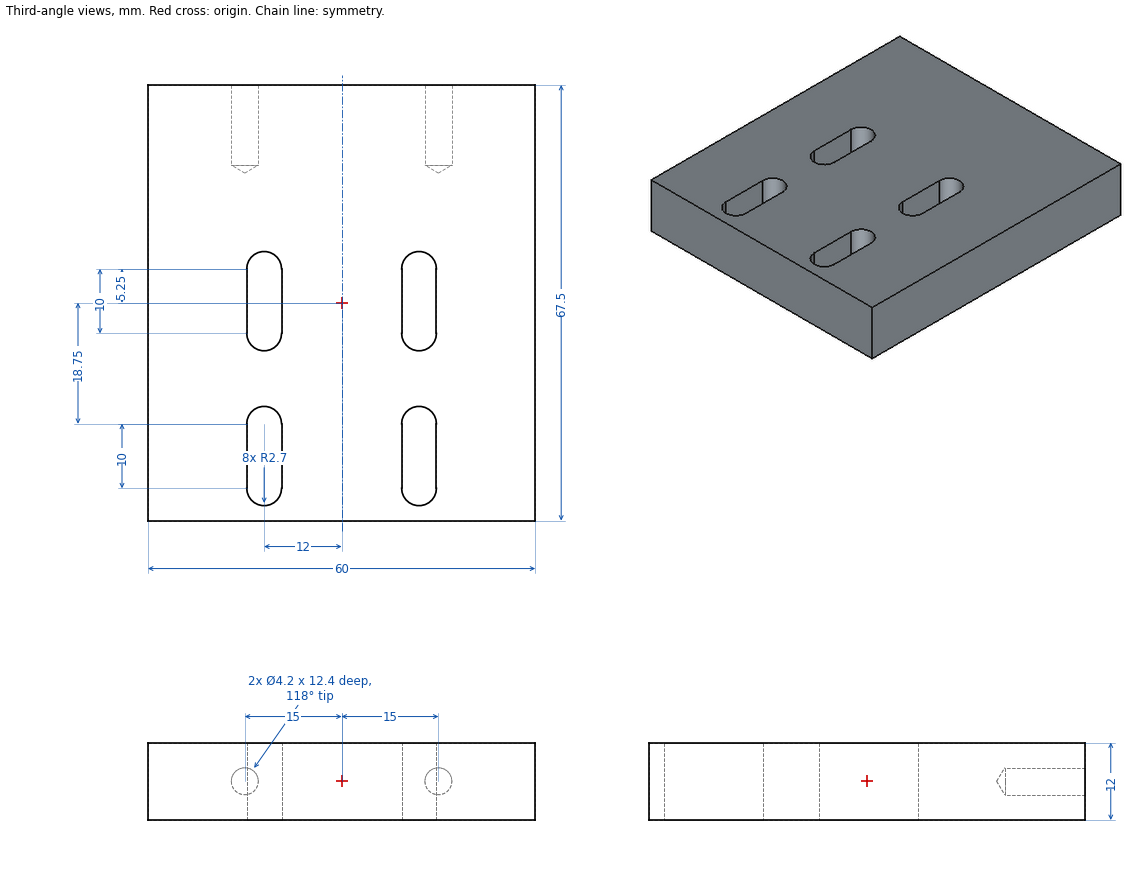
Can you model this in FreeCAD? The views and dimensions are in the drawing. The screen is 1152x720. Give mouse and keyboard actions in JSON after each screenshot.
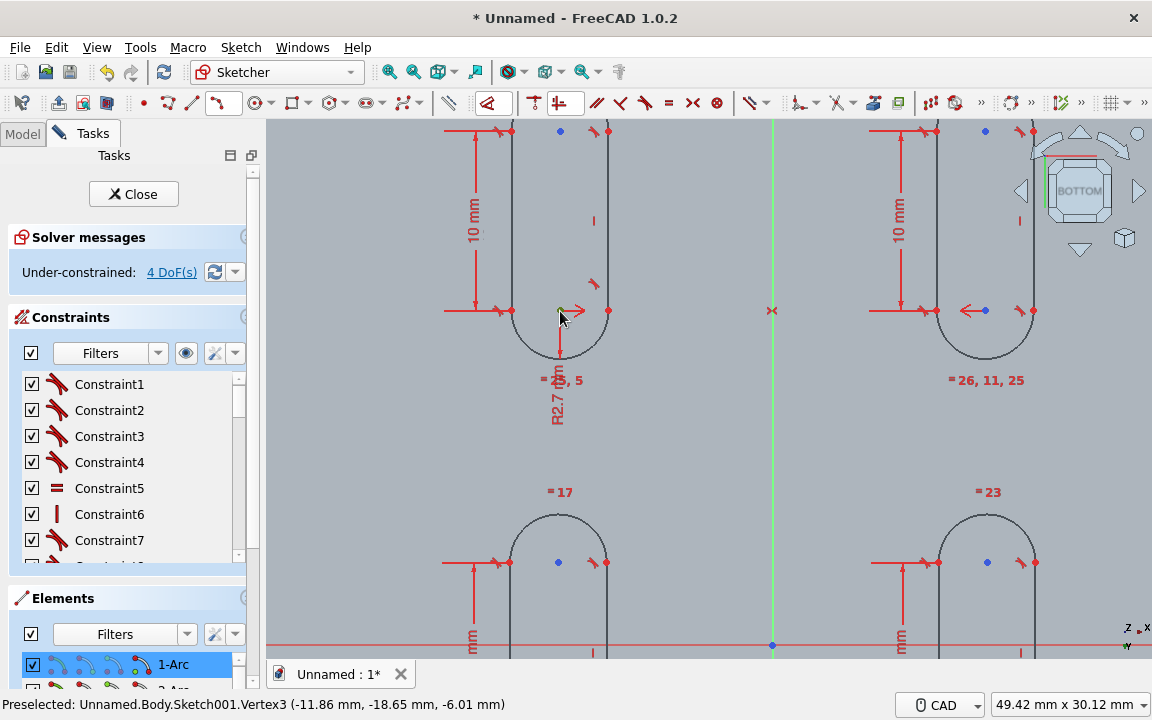
{"action": "key", "text": "l"}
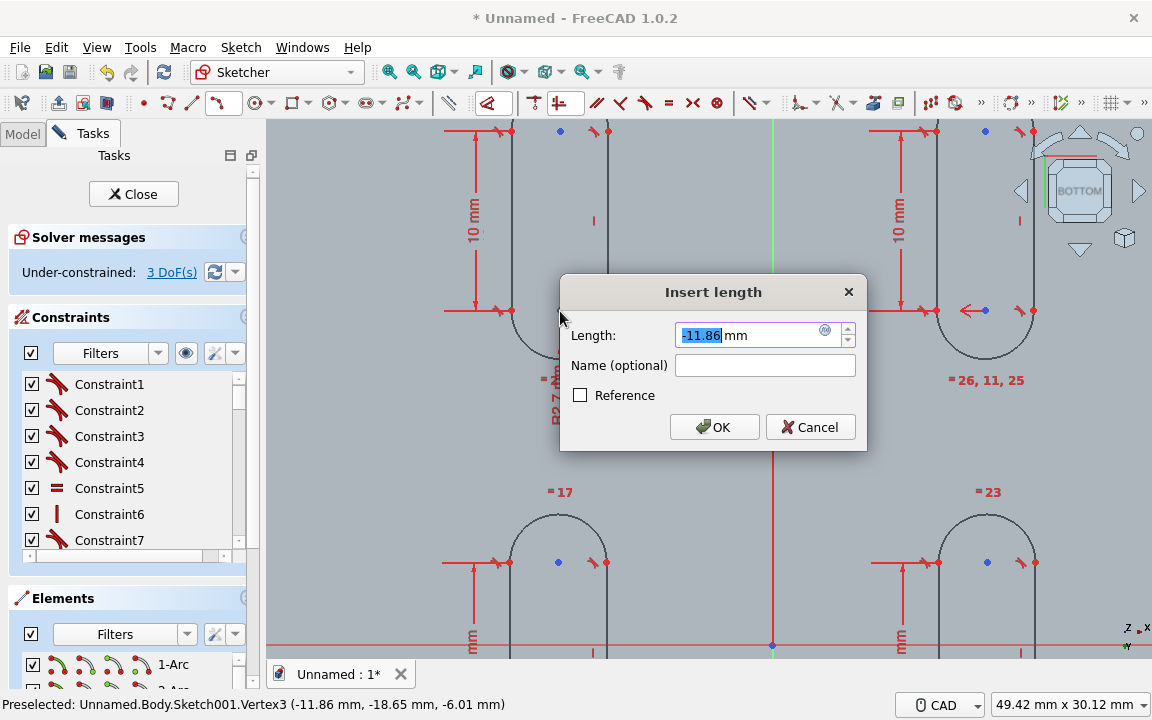
{"action": "type", "text": "-12"}
{"action": "key", "text": "Return"}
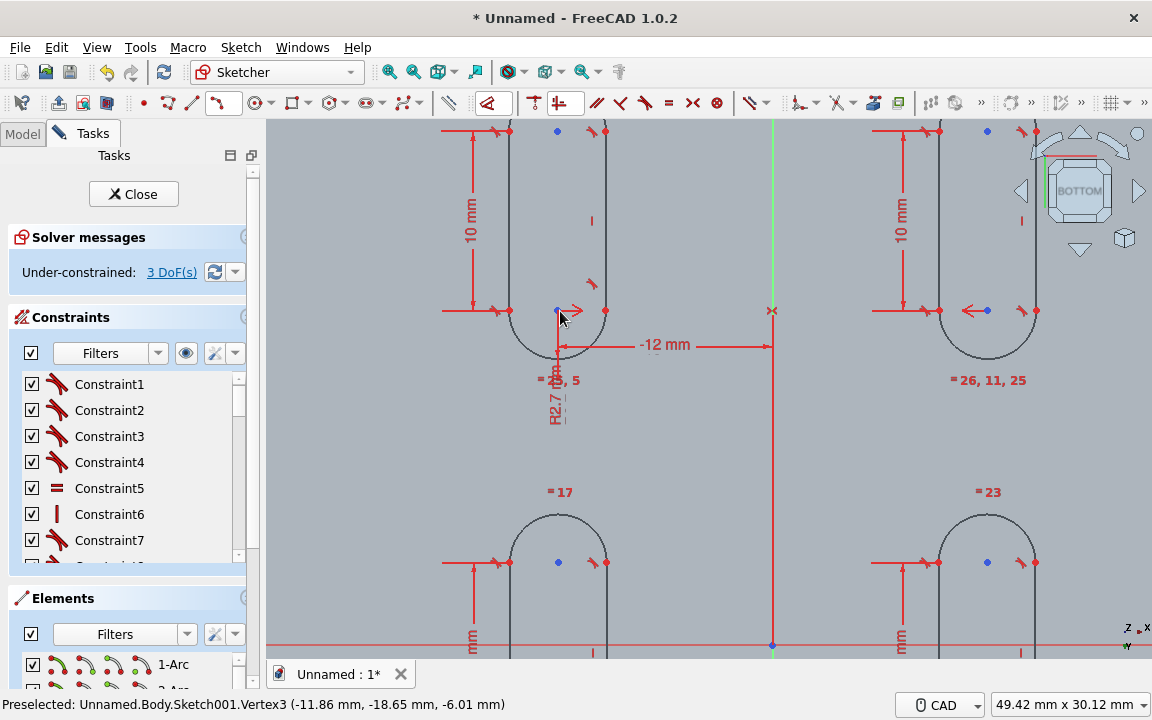
{"action": "scroll", "coordinate": [533, 352], "scroll_direction": "down", "scroll_amount": 4}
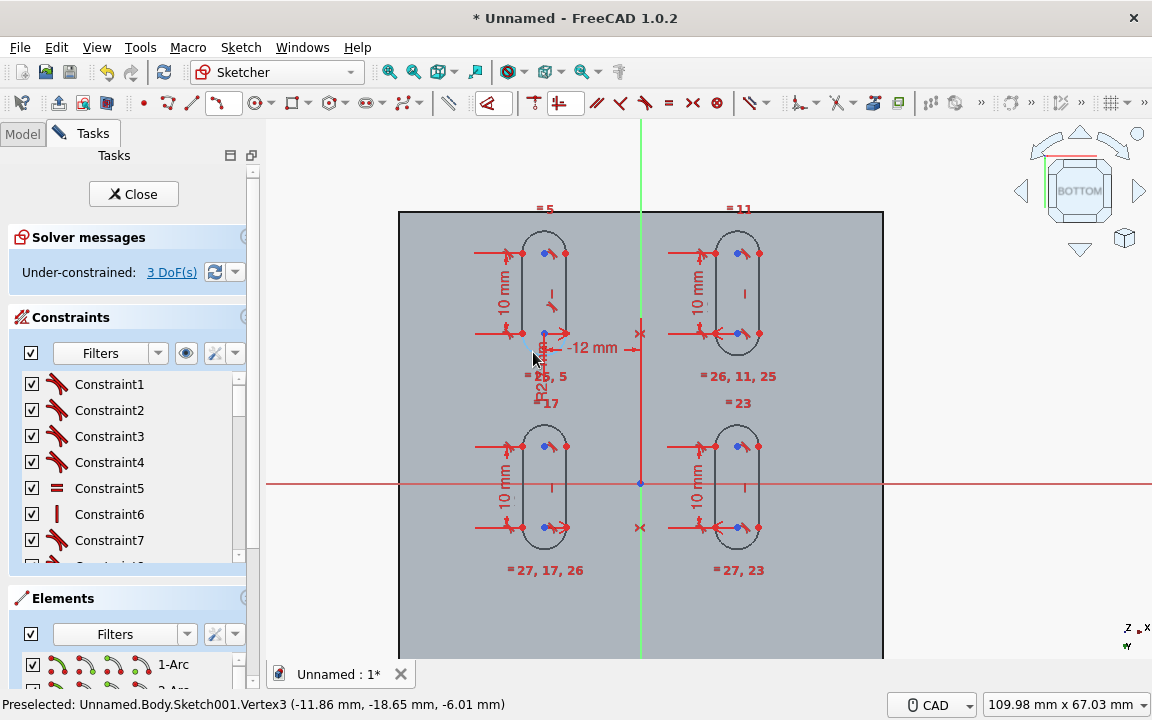
{"action": "left_click", "coordinate": [545, 528]}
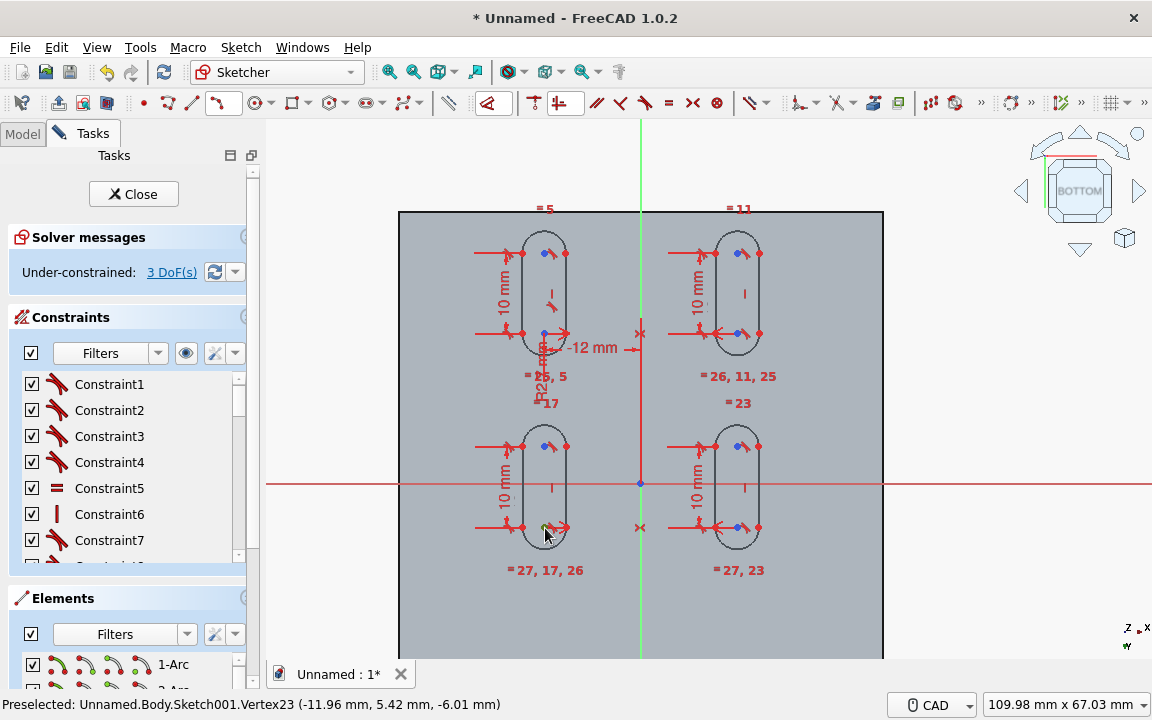
{"action": "key", "text": "l"}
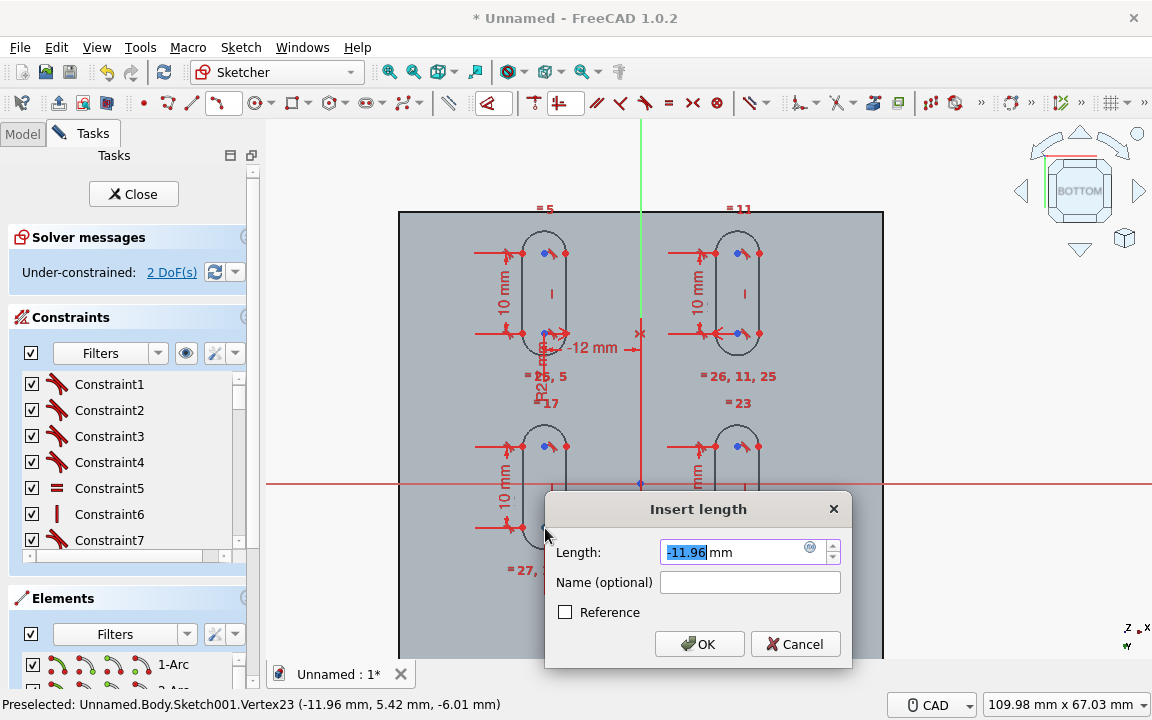
{"action": "type", "text": "-12"}
{"action": "key", "text": "Return"}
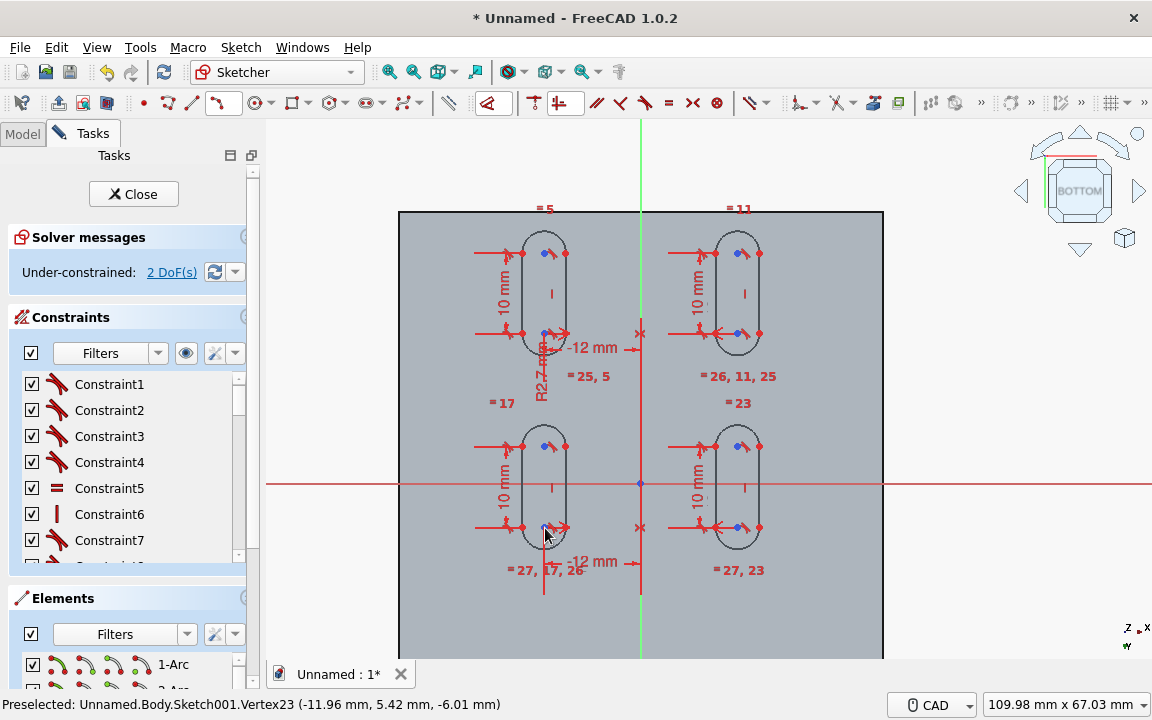
{"action": "left_click", "coordinate": [522, 528]}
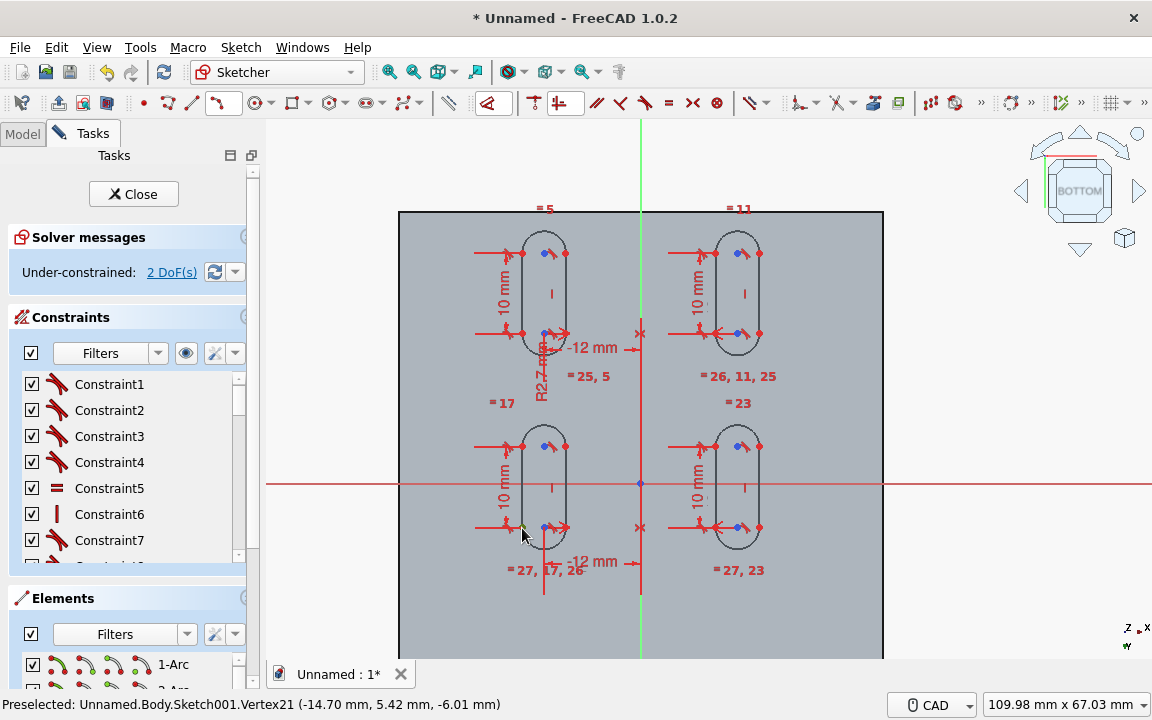
{"action": "key", "text": "i"}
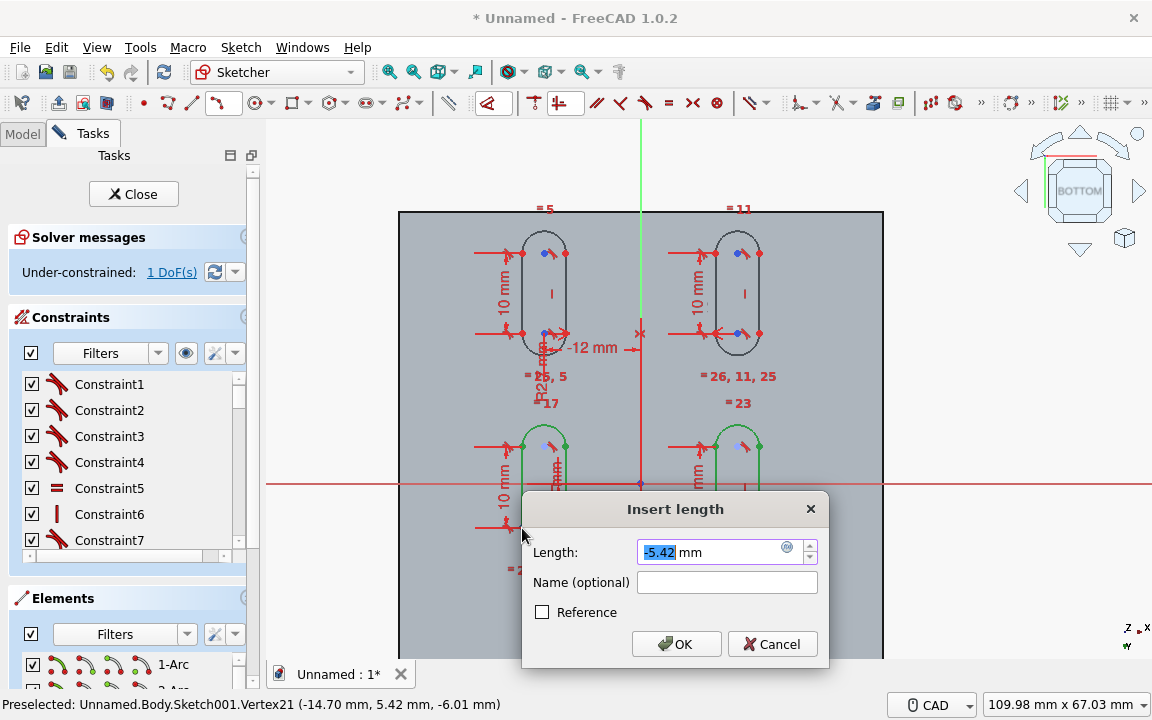
{"action": "type", "text": "-5.25"}
{"action": "key", "text": "Return"}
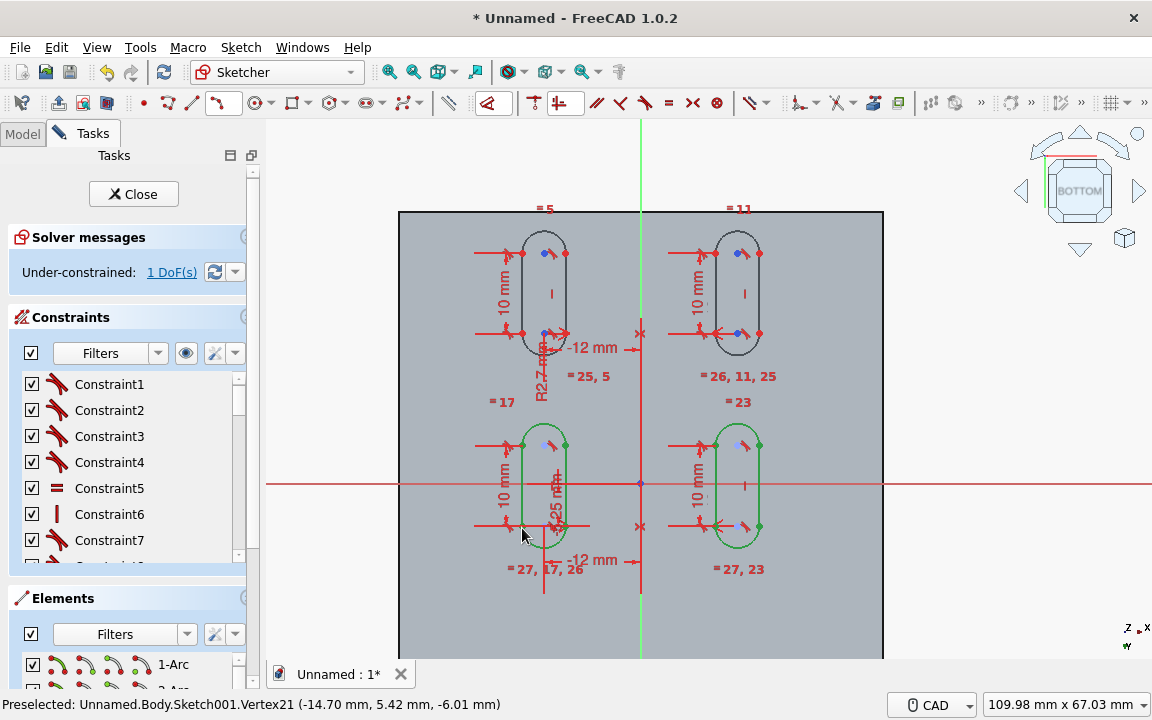
{"action": "left_click", "coordinate": [522, 334]}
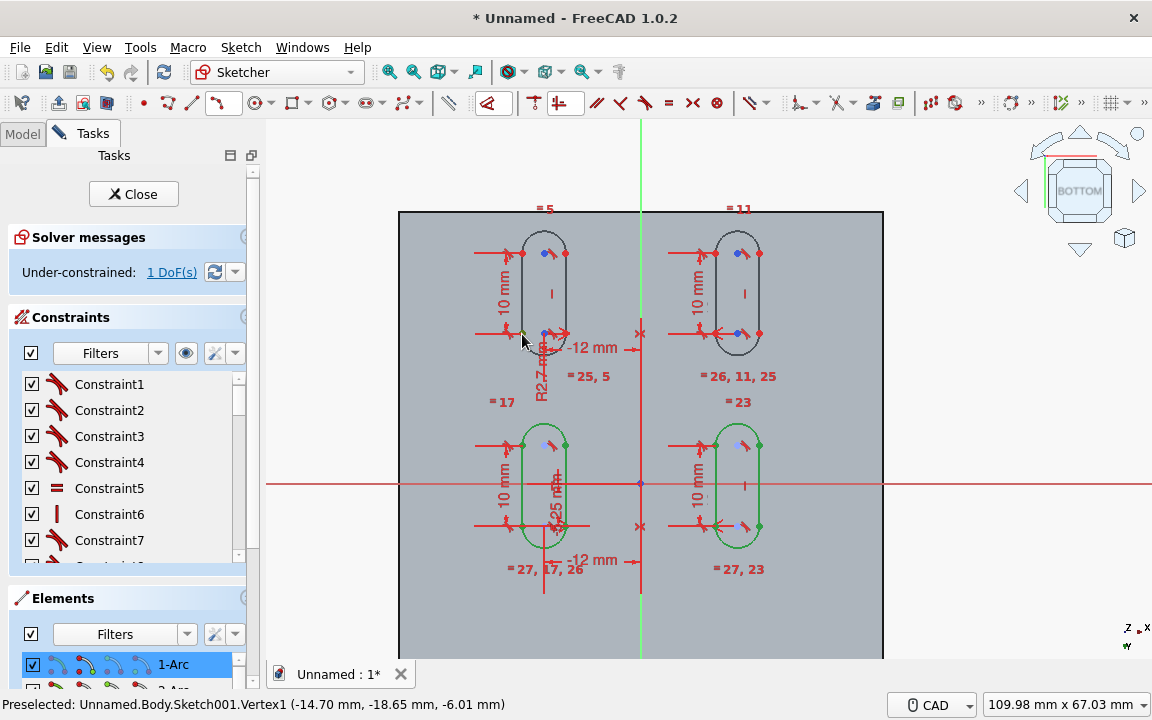
{"action": "key", "text": "i"}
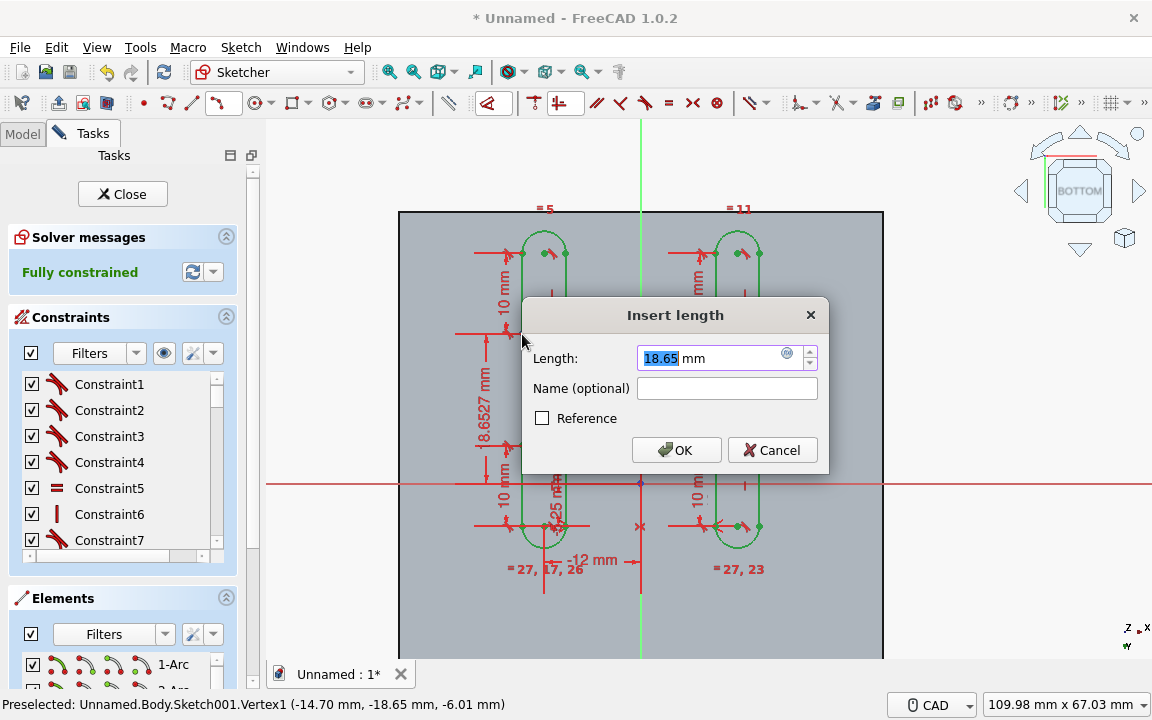
{"action": "type", "text": "18.75"}
{"action": "key", "text": "Return"}